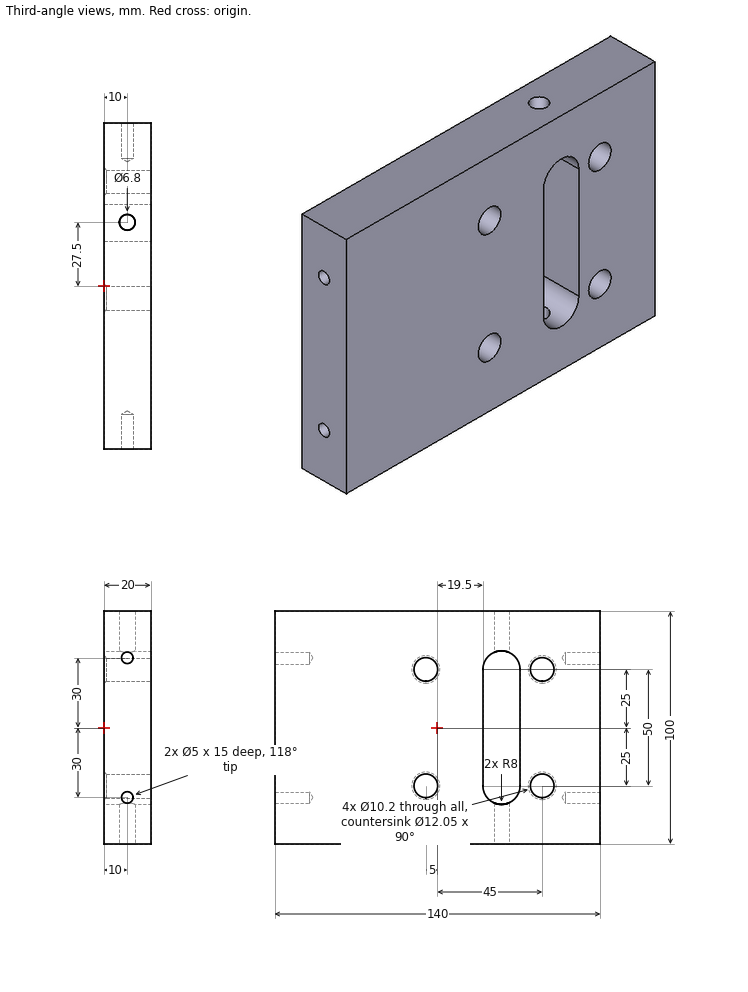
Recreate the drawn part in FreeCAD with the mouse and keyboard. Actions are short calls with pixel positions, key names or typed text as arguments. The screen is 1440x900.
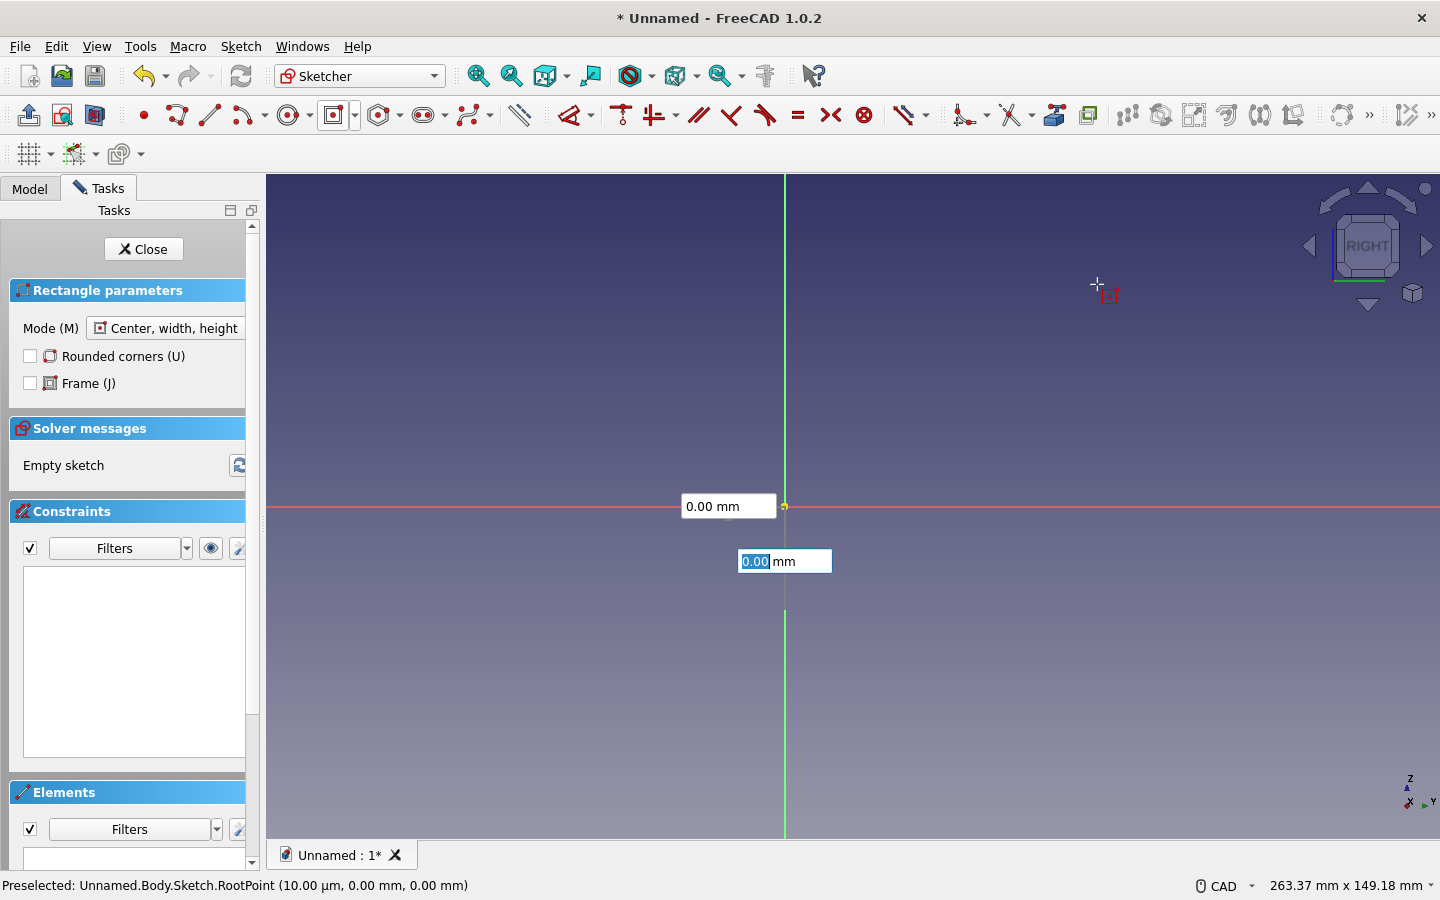
text(140)
key(Tab)
text(100)
key(Return)
key(Escape)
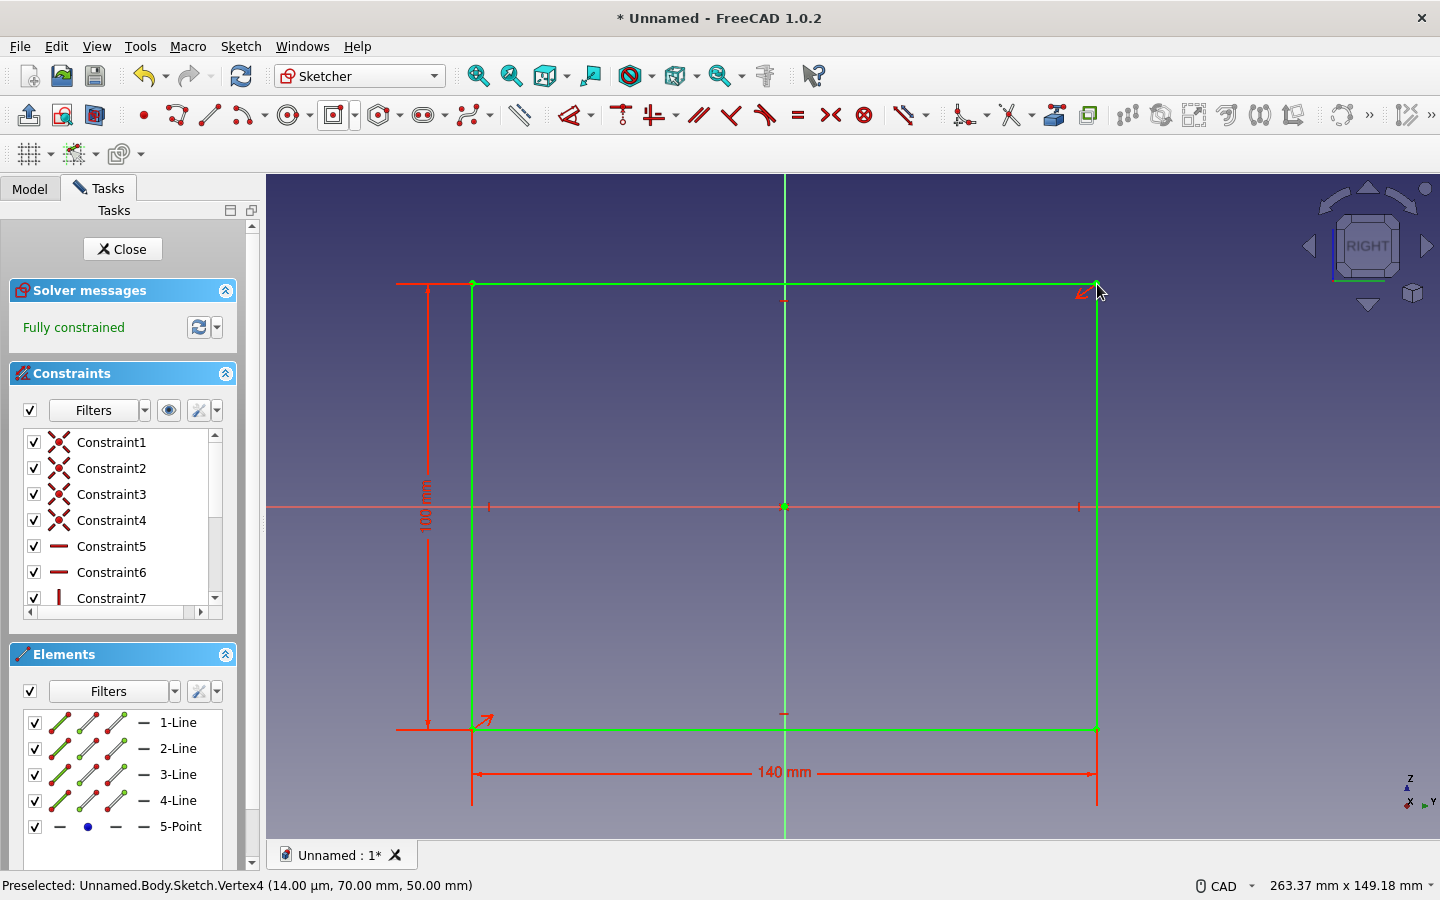
click(123, 249)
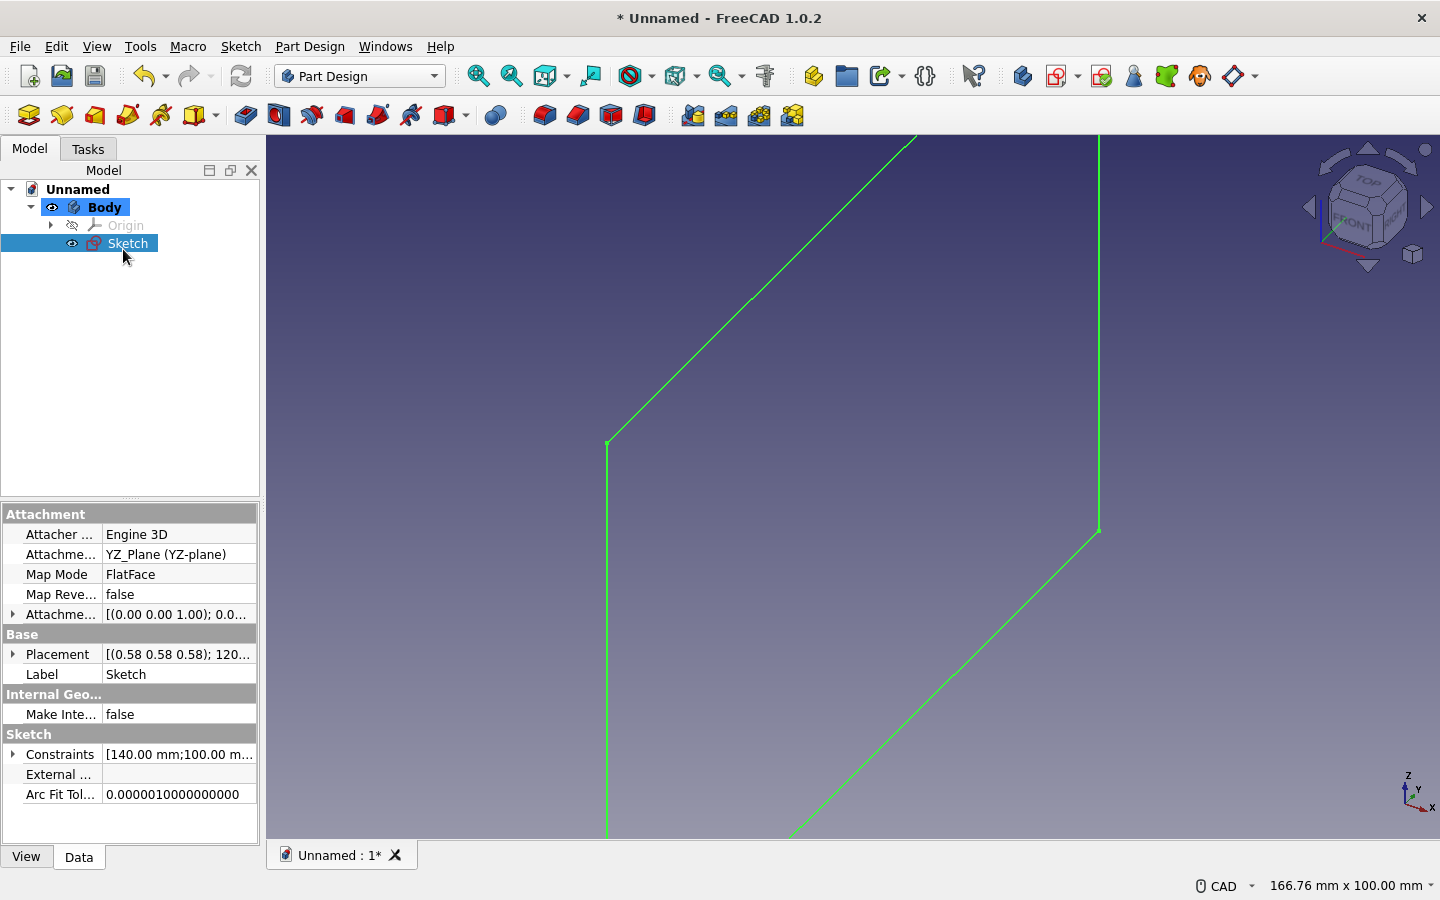
click(29, 116)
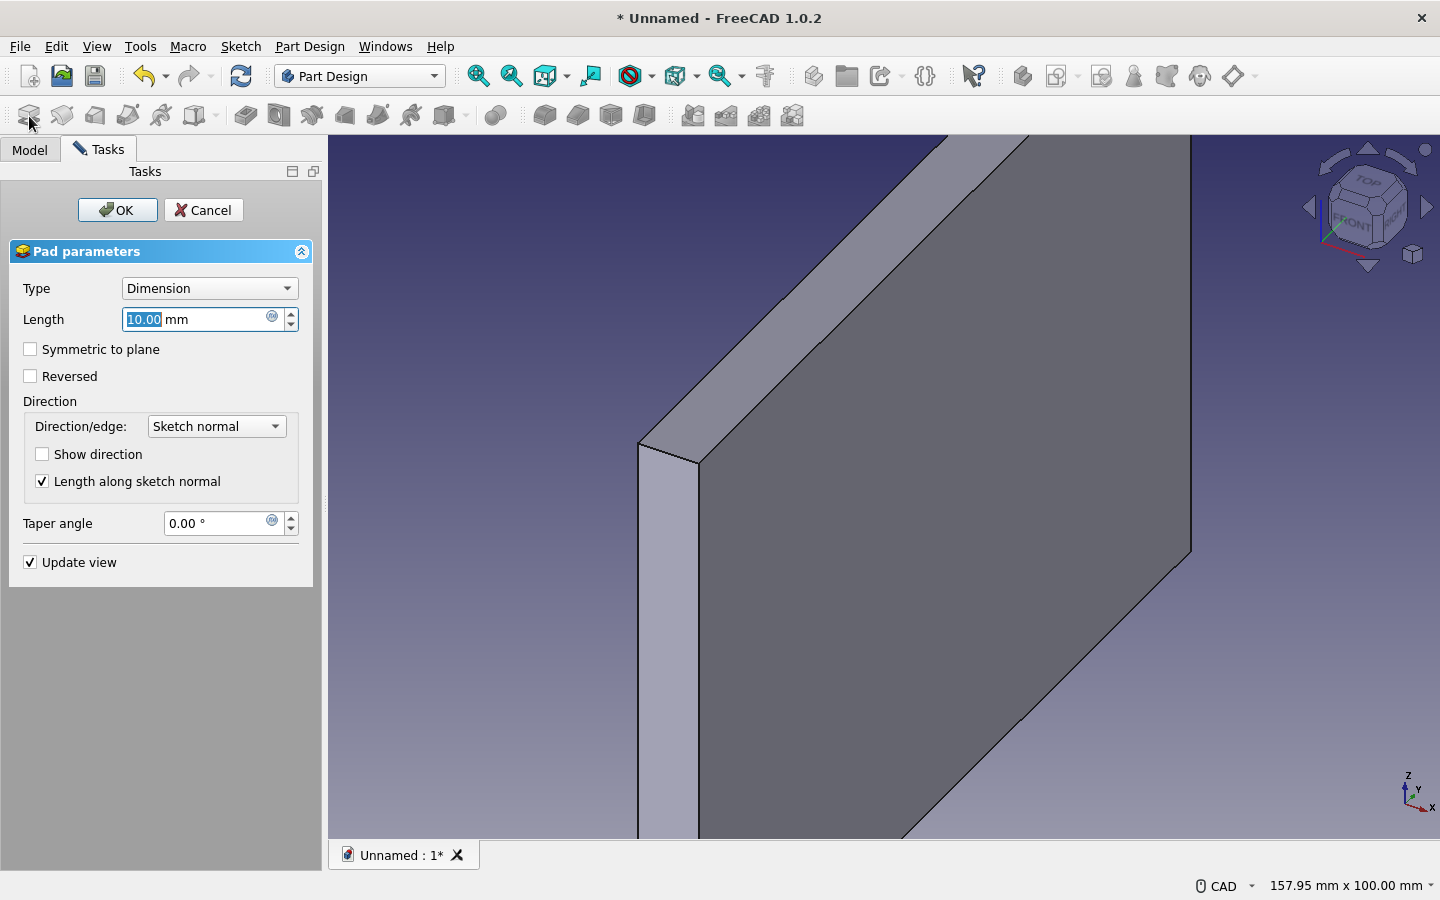
text(20)
key(Tab)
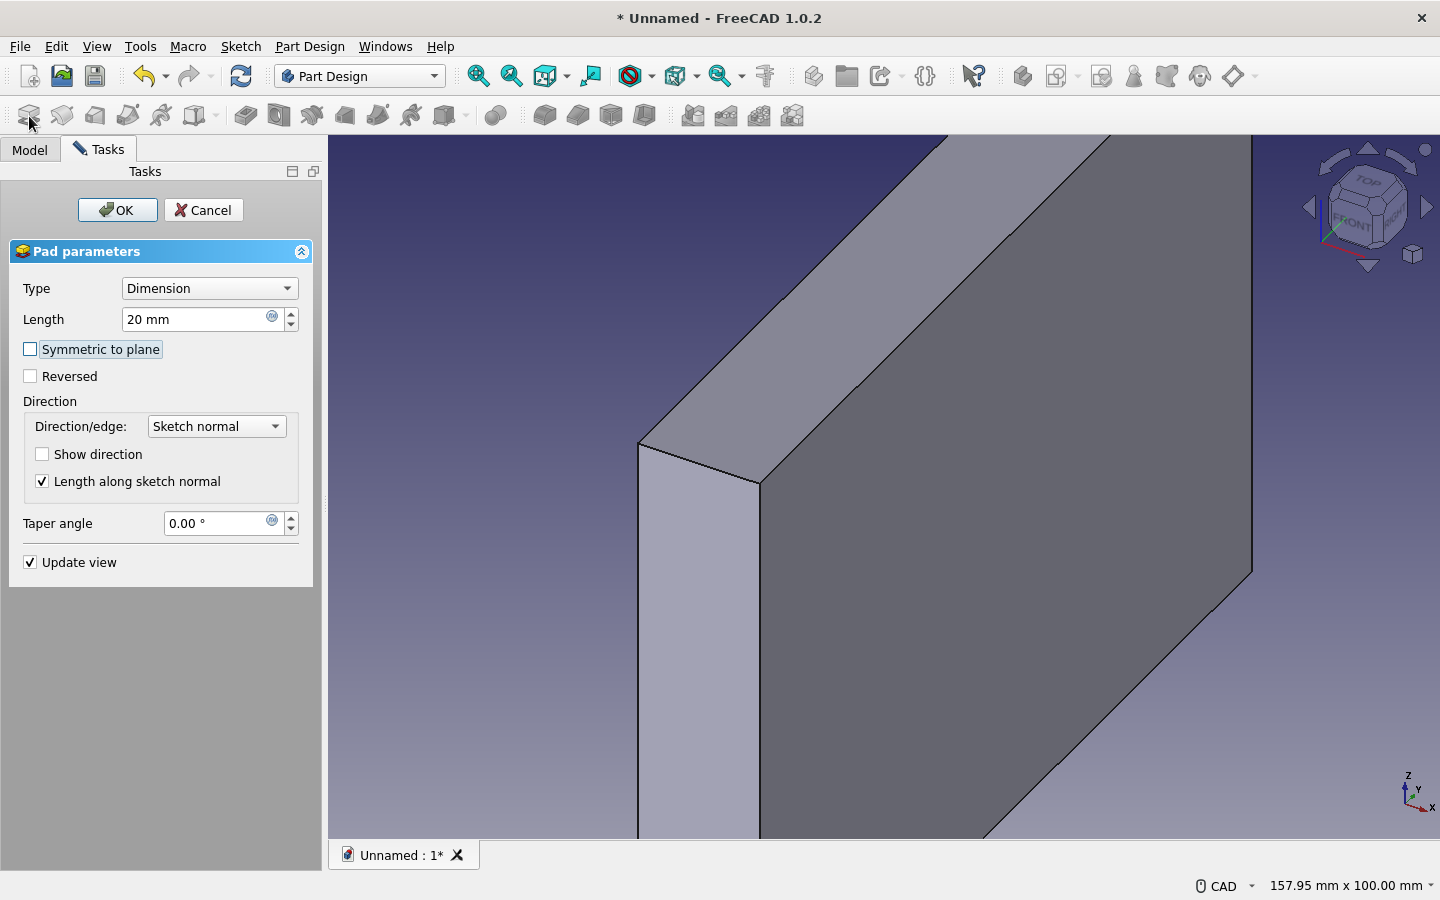
click(118, 210)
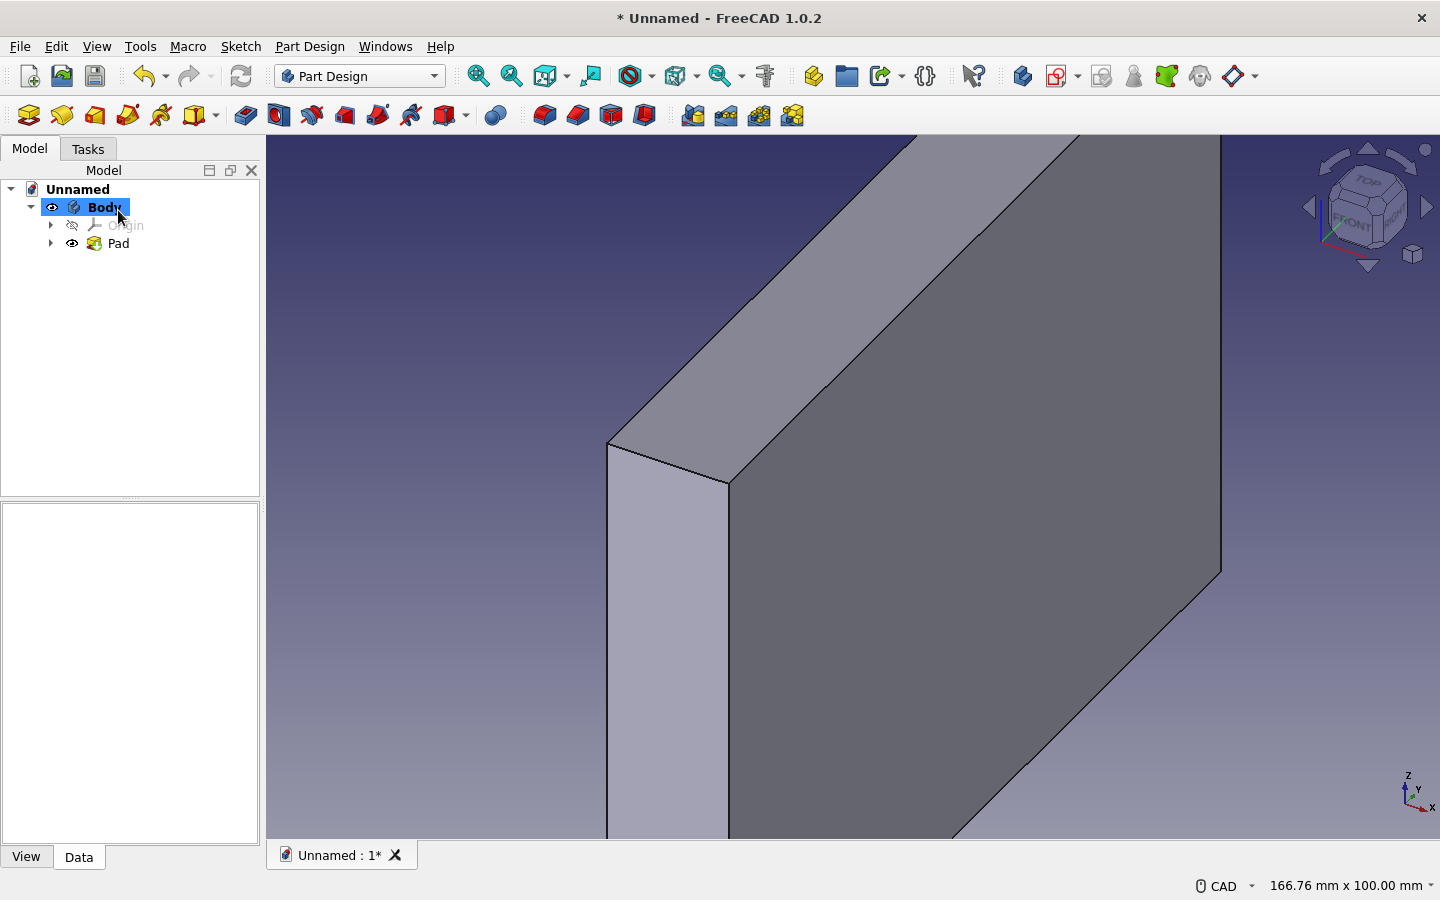
click(479, 76)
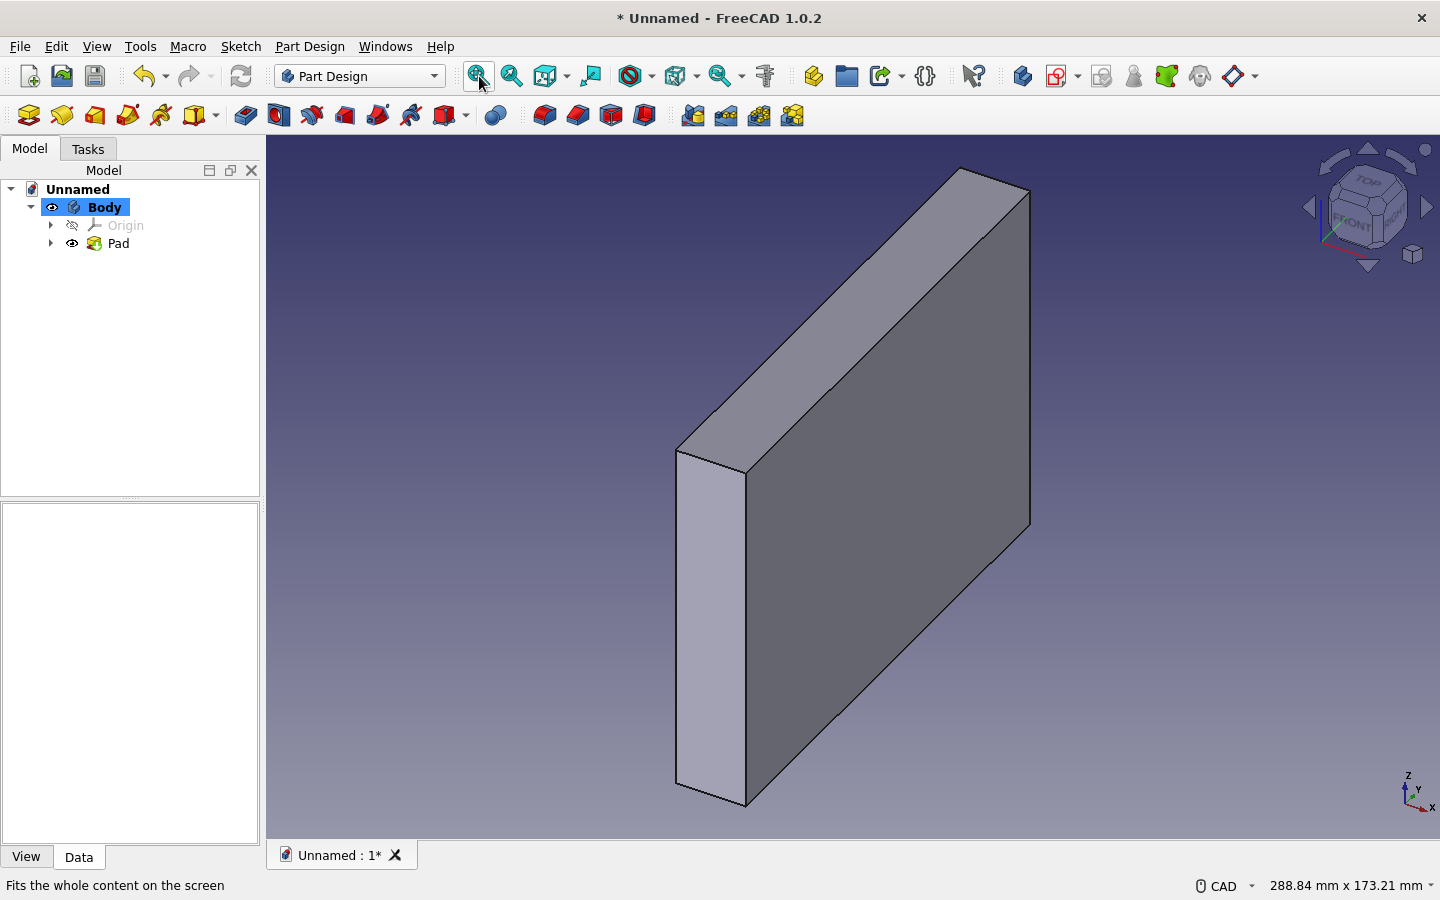
click(711, 627)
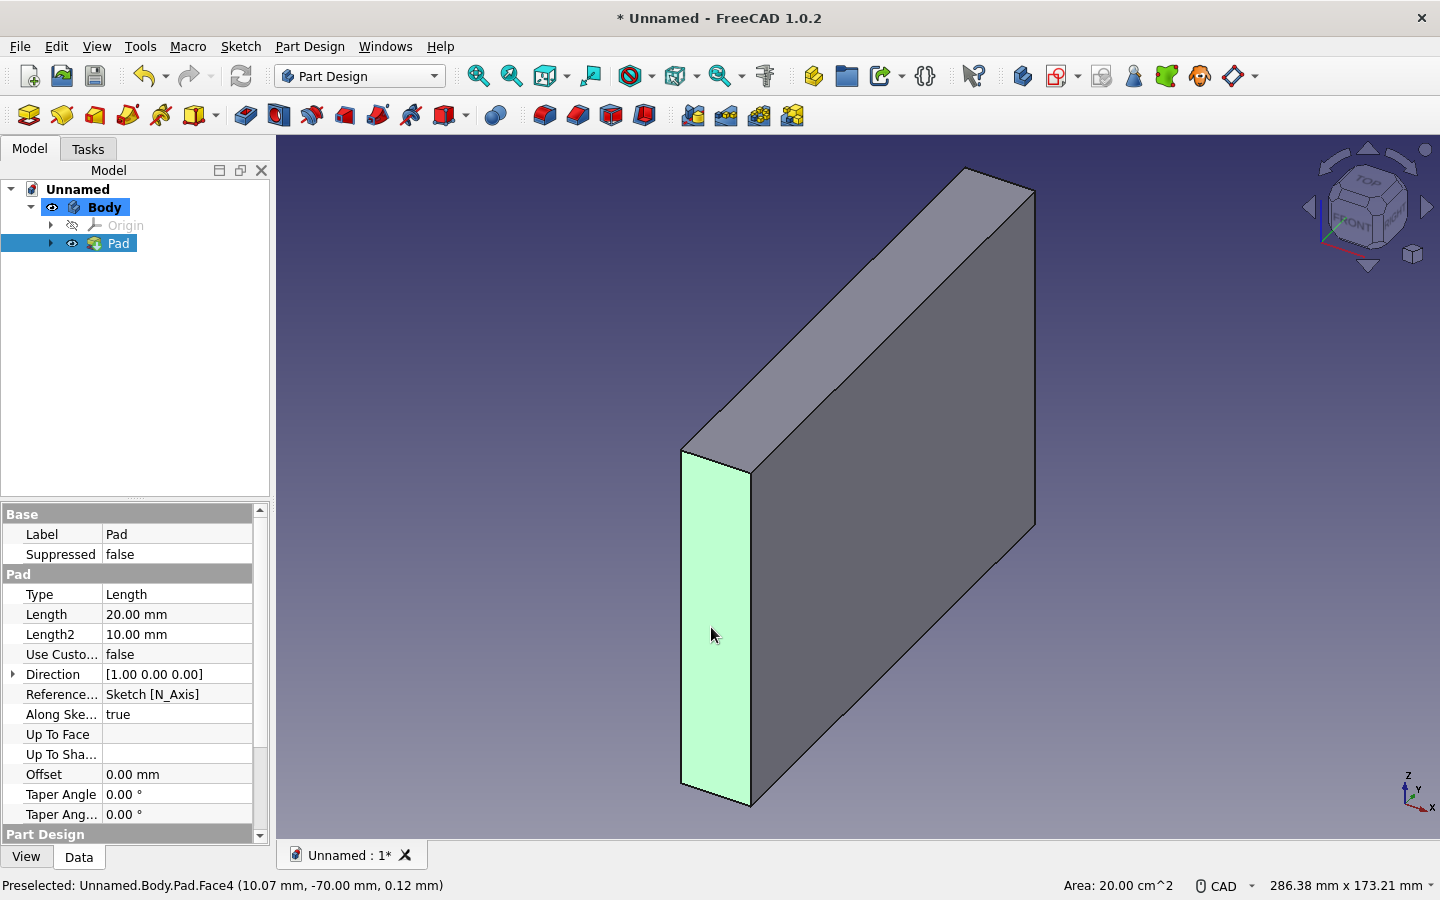
click(1056, 76)